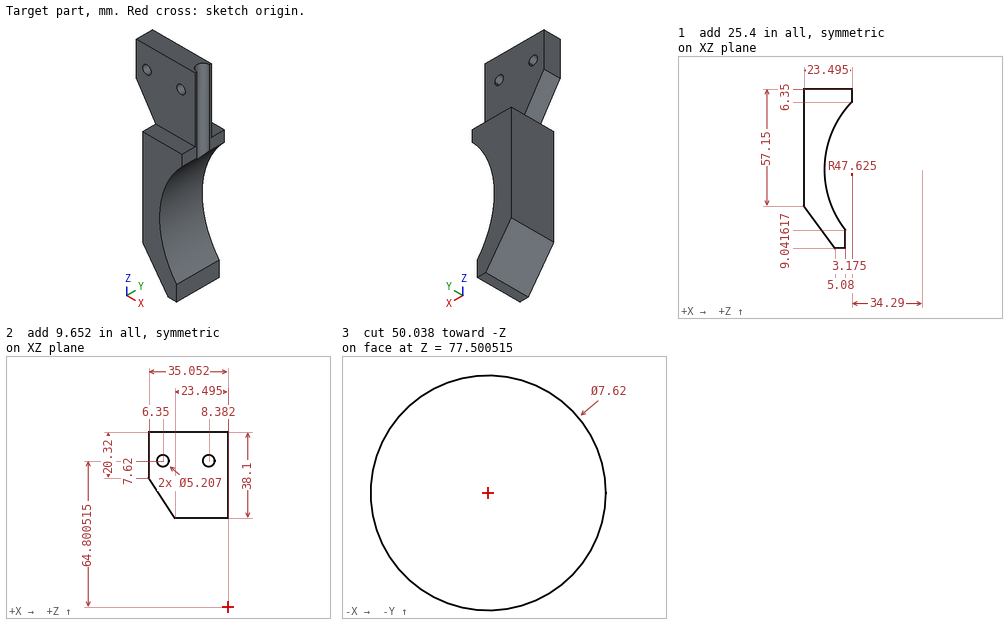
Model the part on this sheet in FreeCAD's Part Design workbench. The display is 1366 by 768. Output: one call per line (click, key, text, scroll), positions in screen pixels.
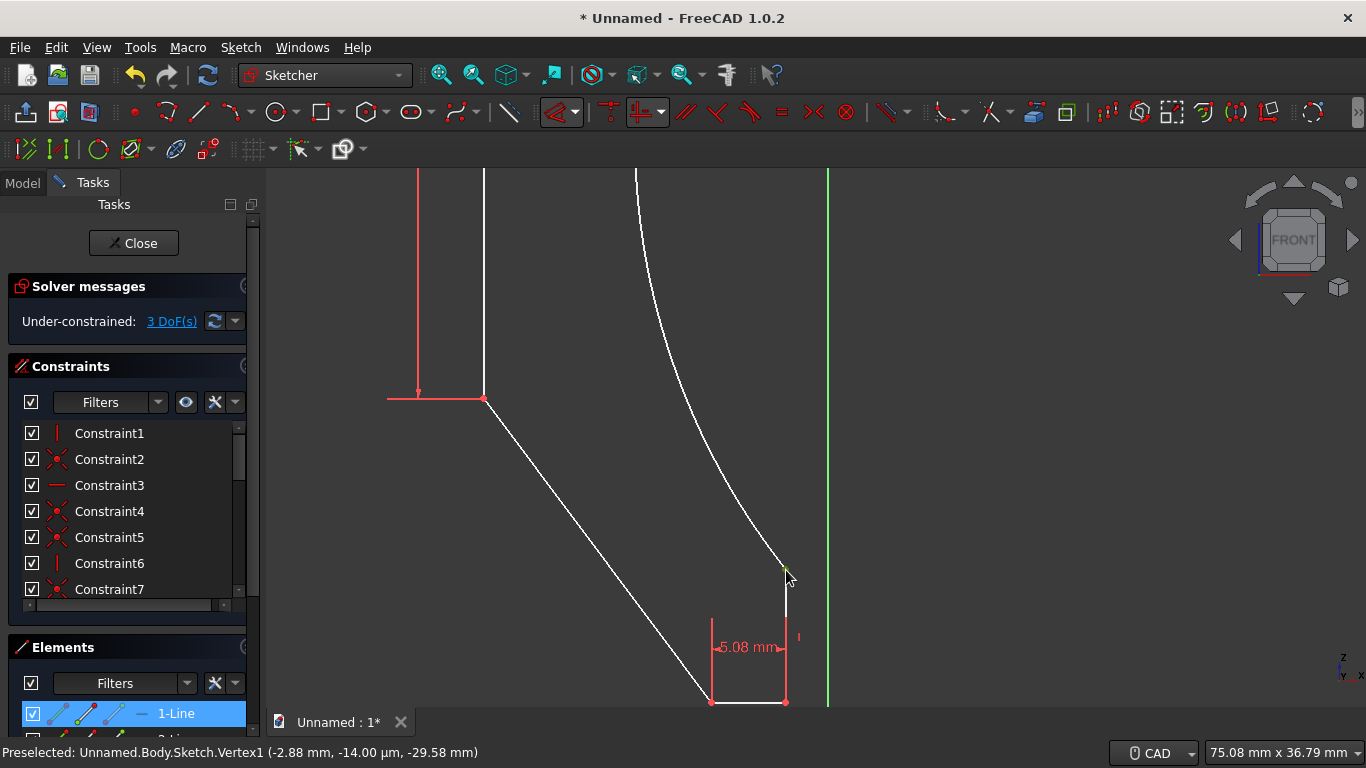
click(578, 112)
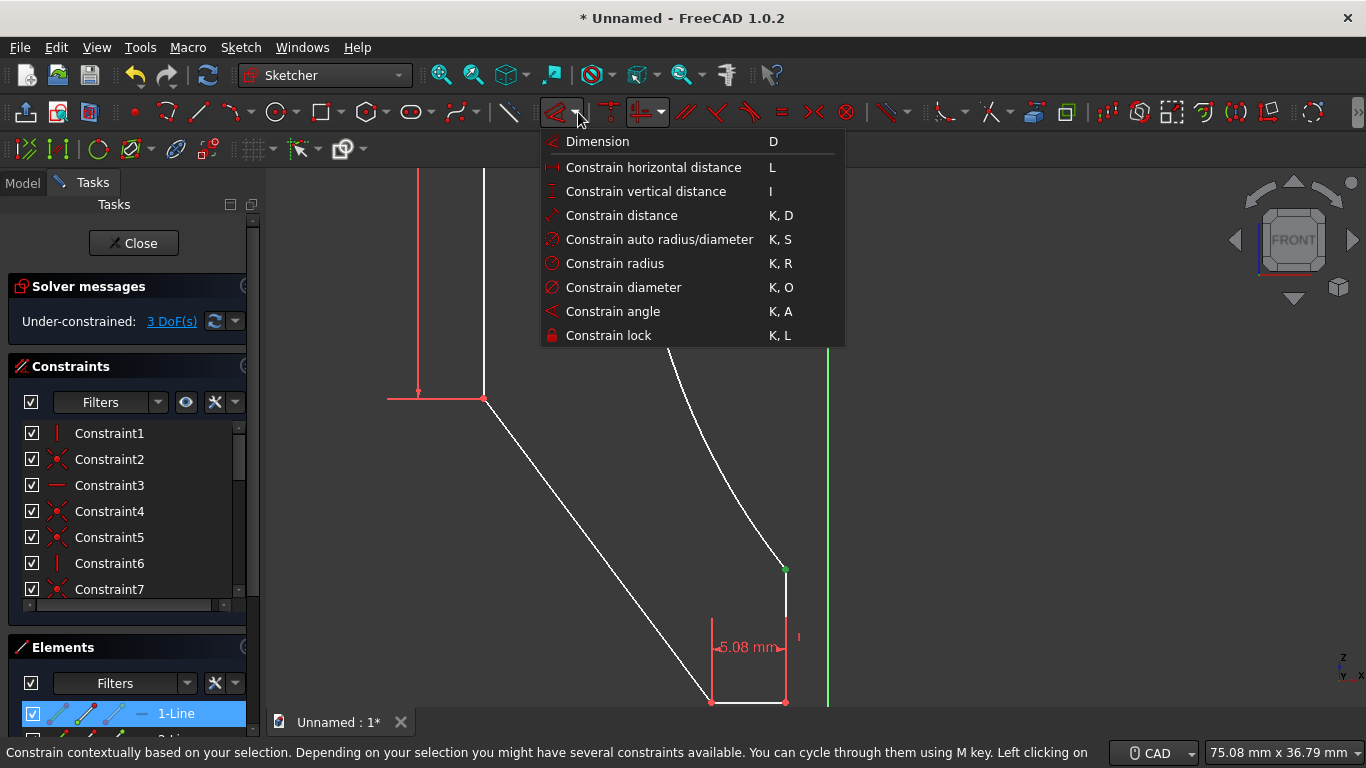
click(693, 167)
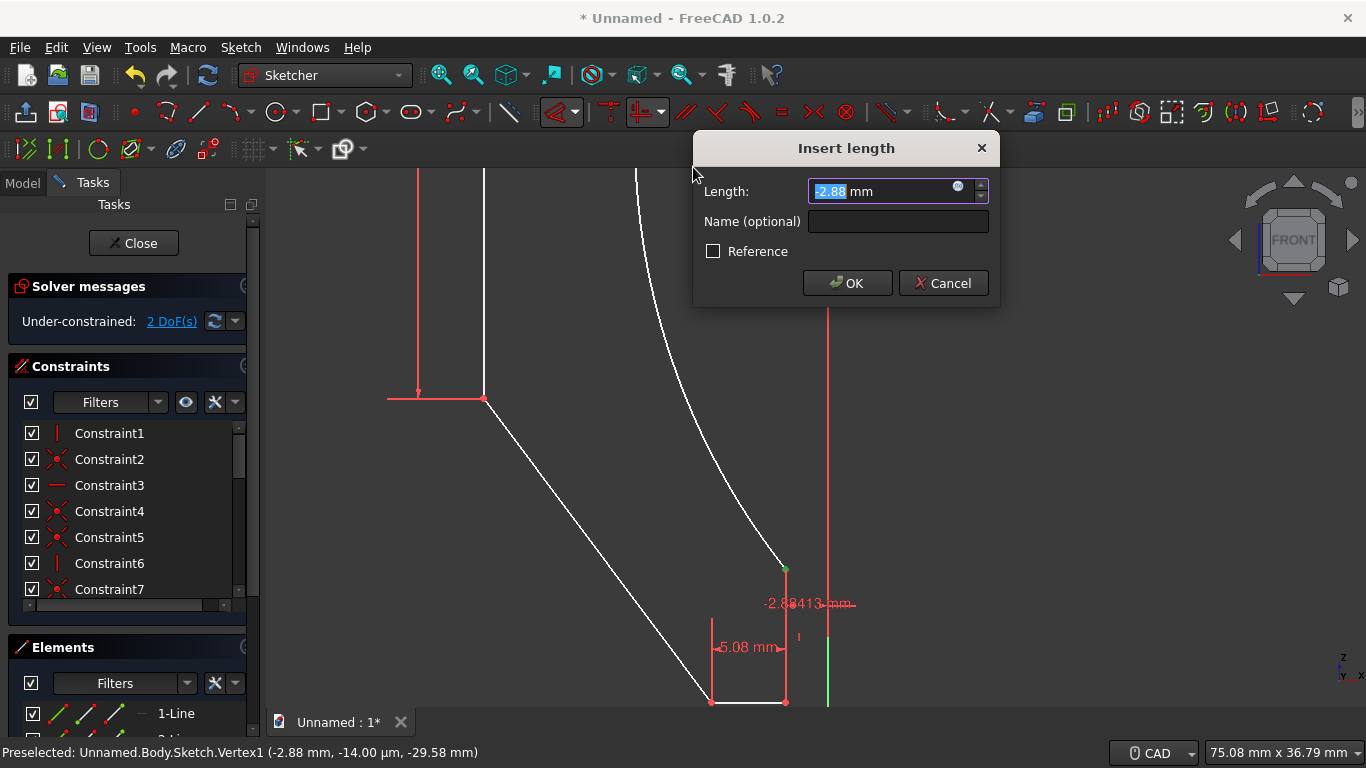
text(-3.175)
key(Return)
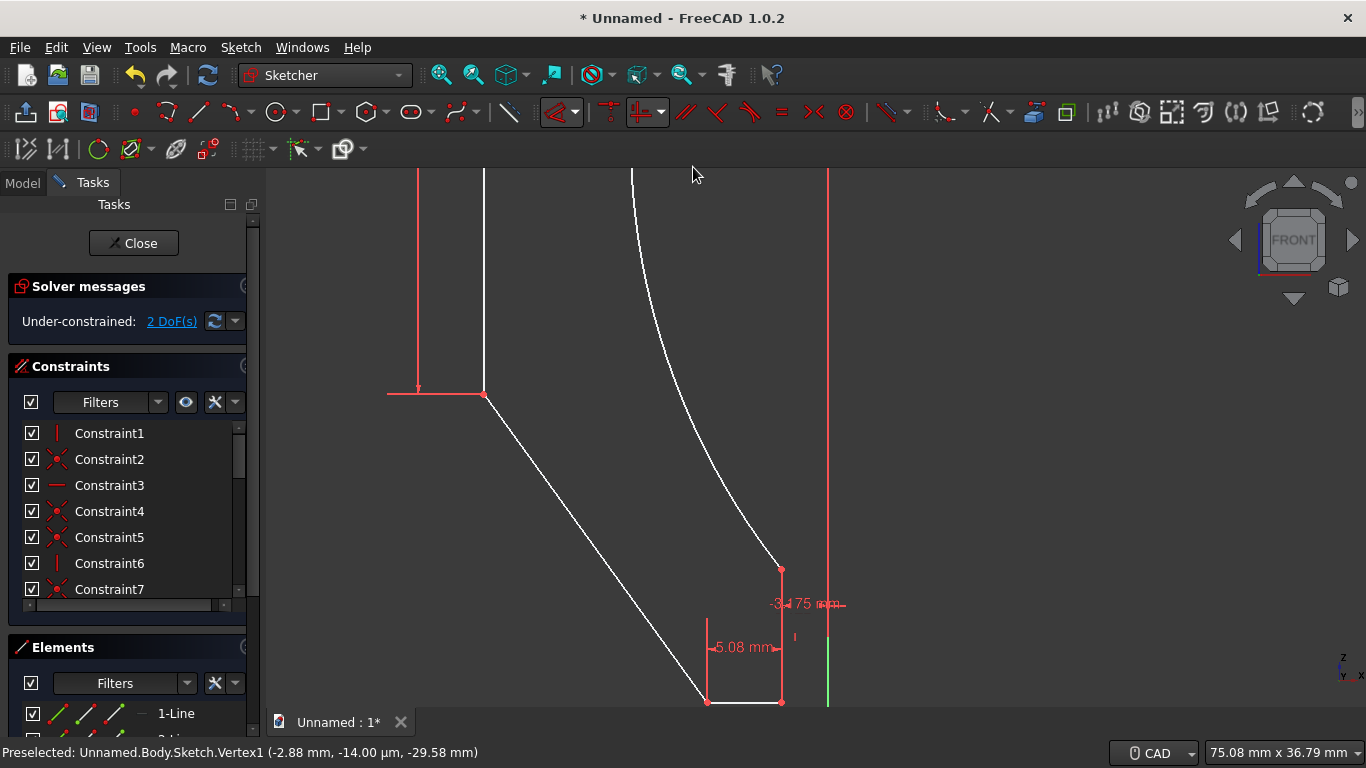
scroll(787, 570, down, 6)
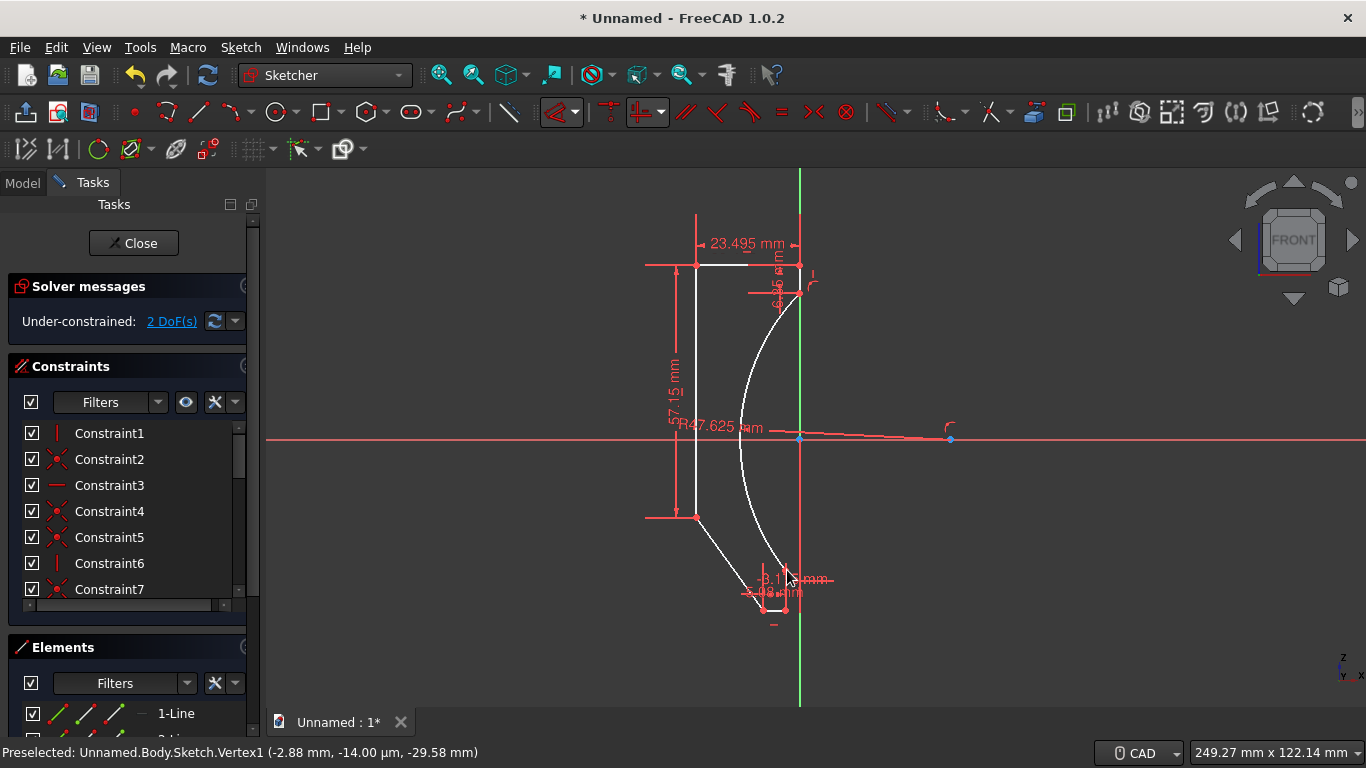
click(950, 440)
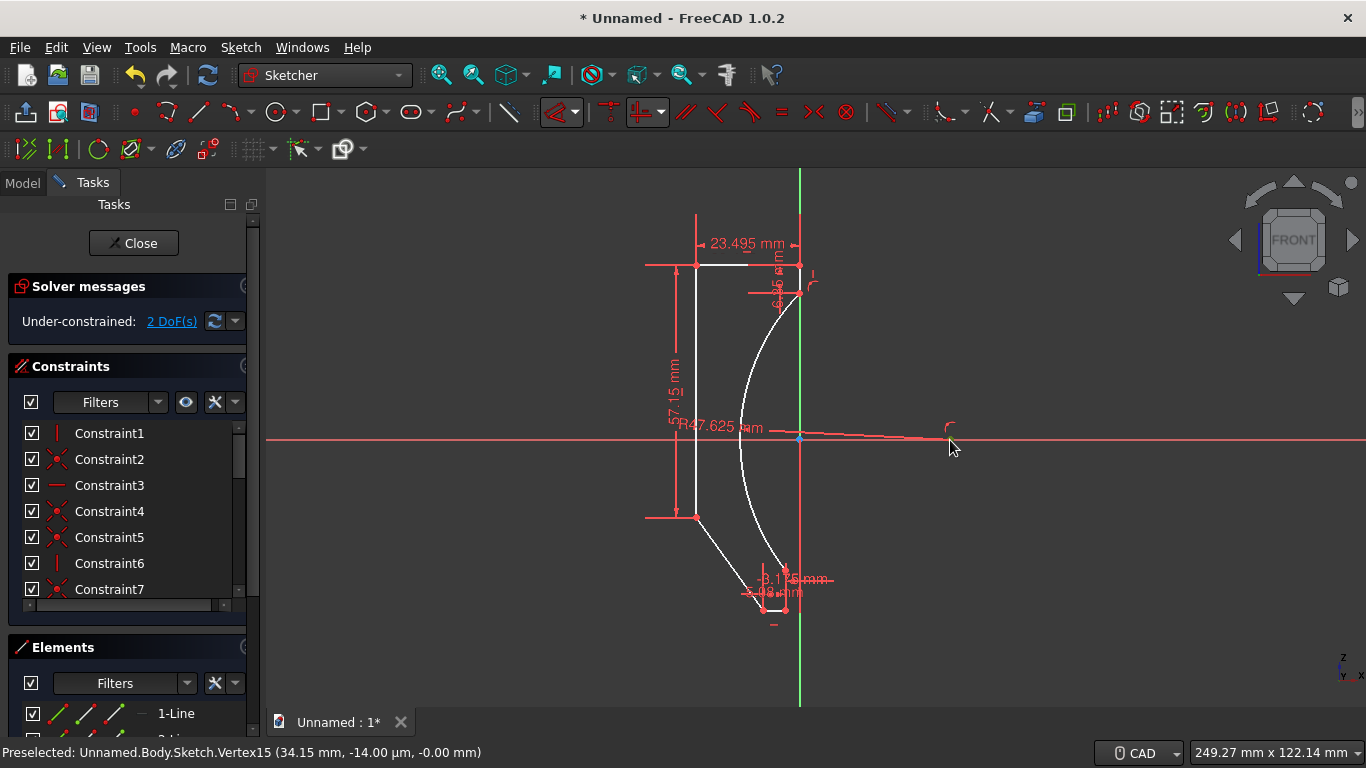
key(l)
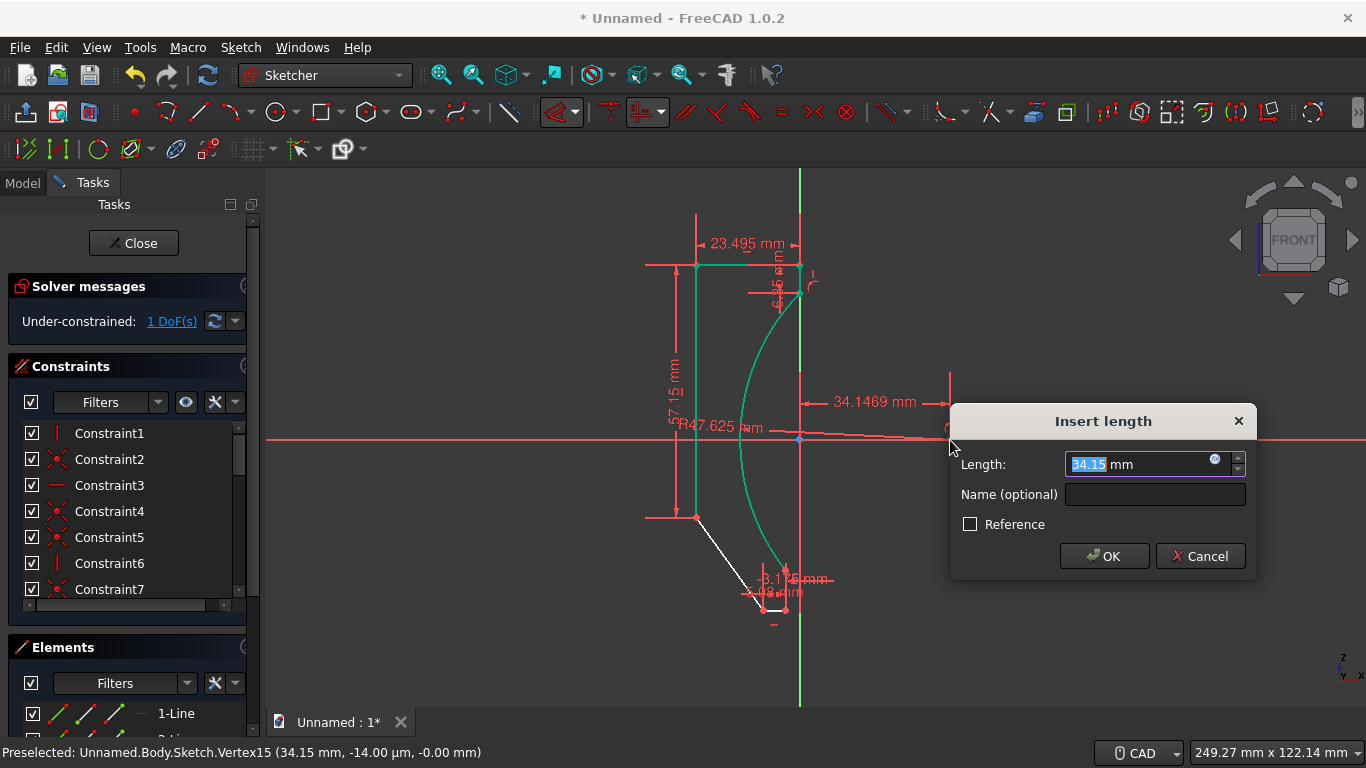
text(34.29)
key(Return)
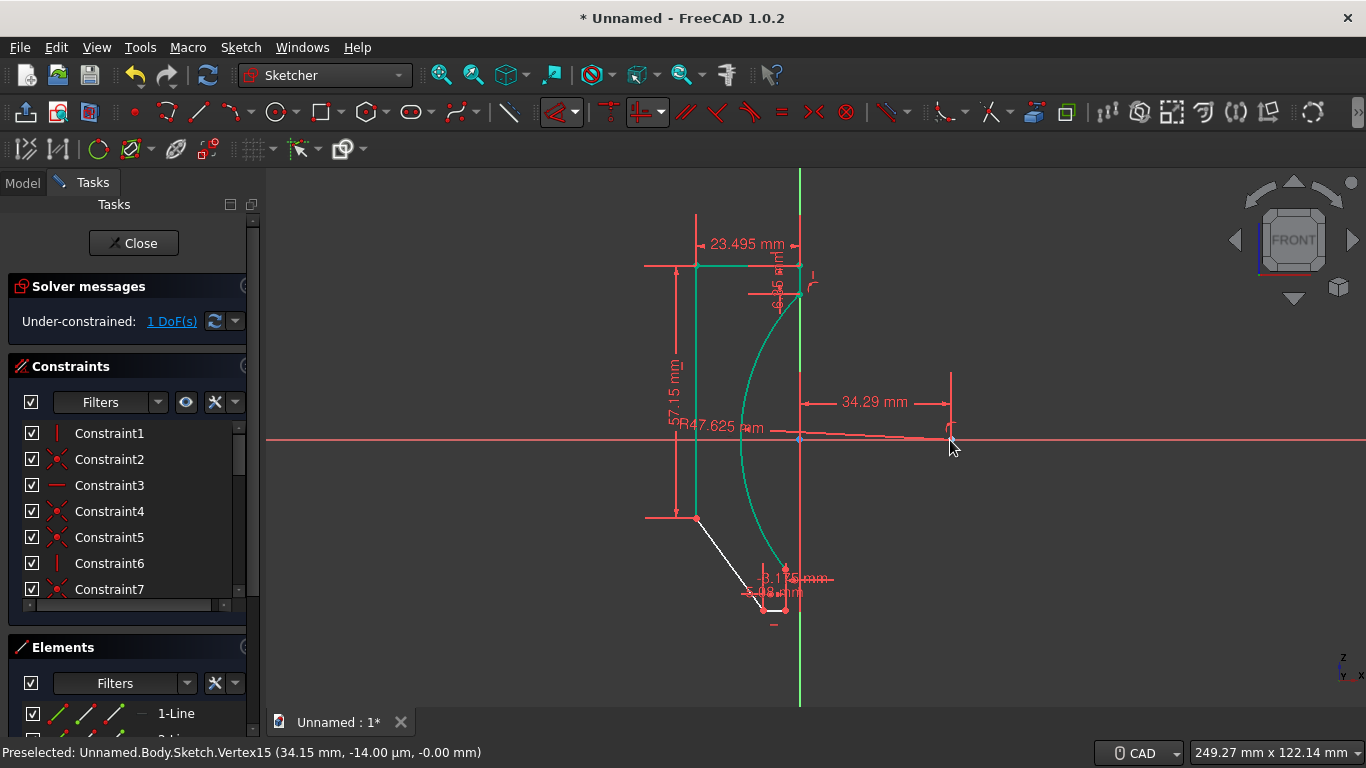
click(786, 602)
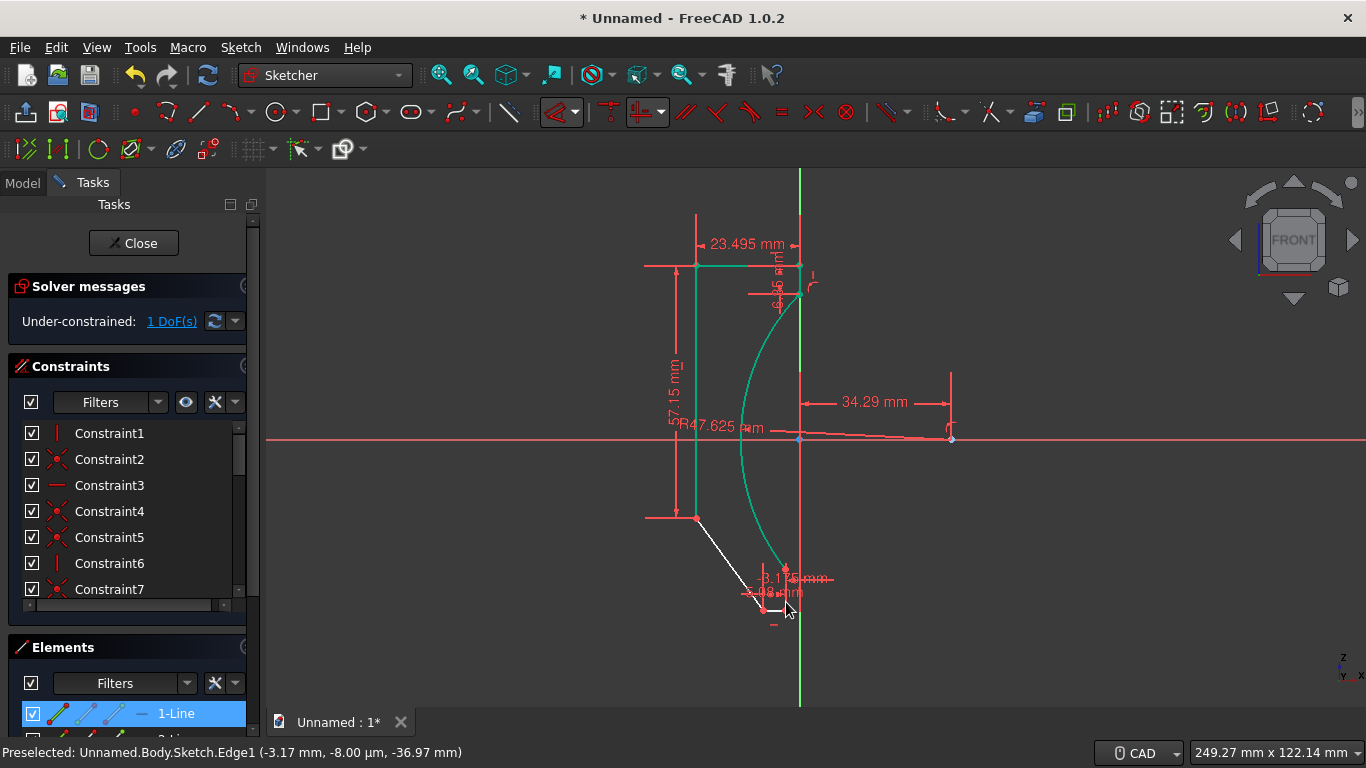
key(i)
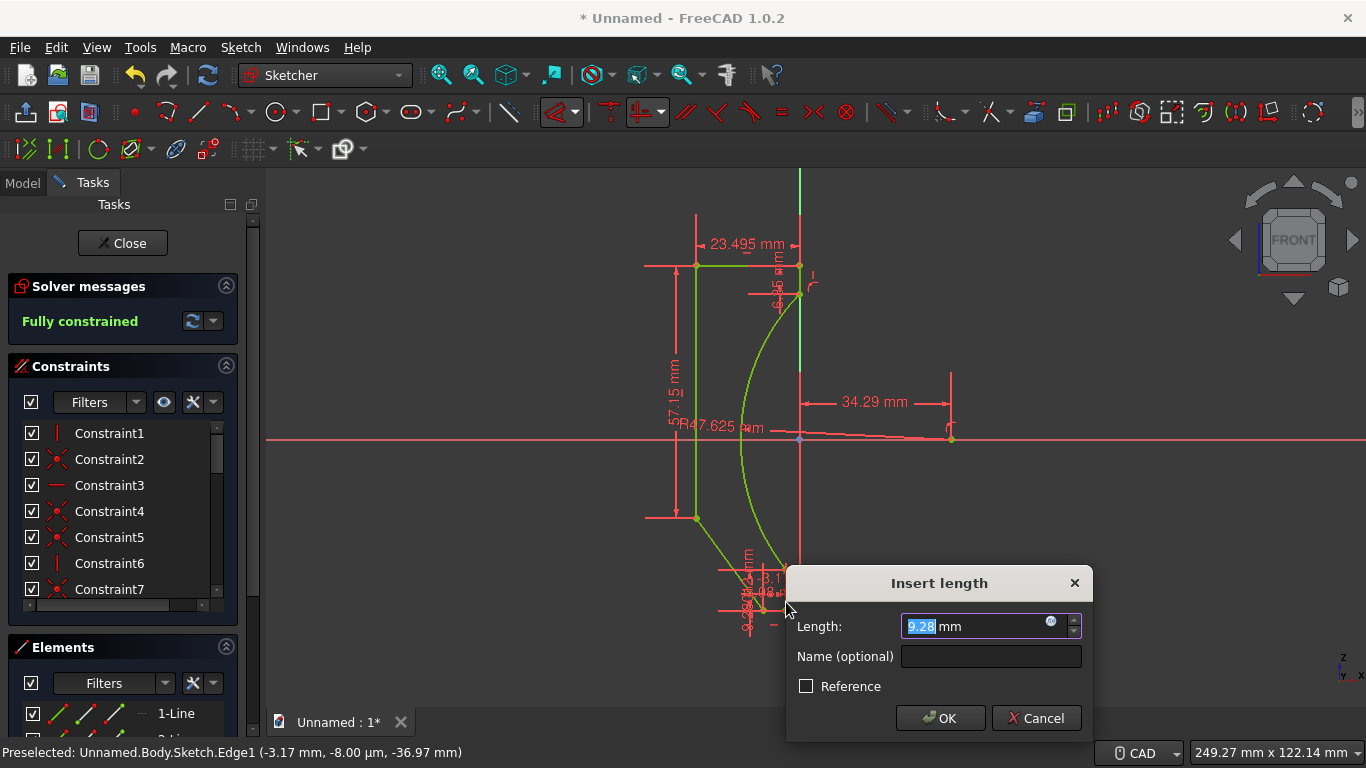
text(9.041617)
key(Return)